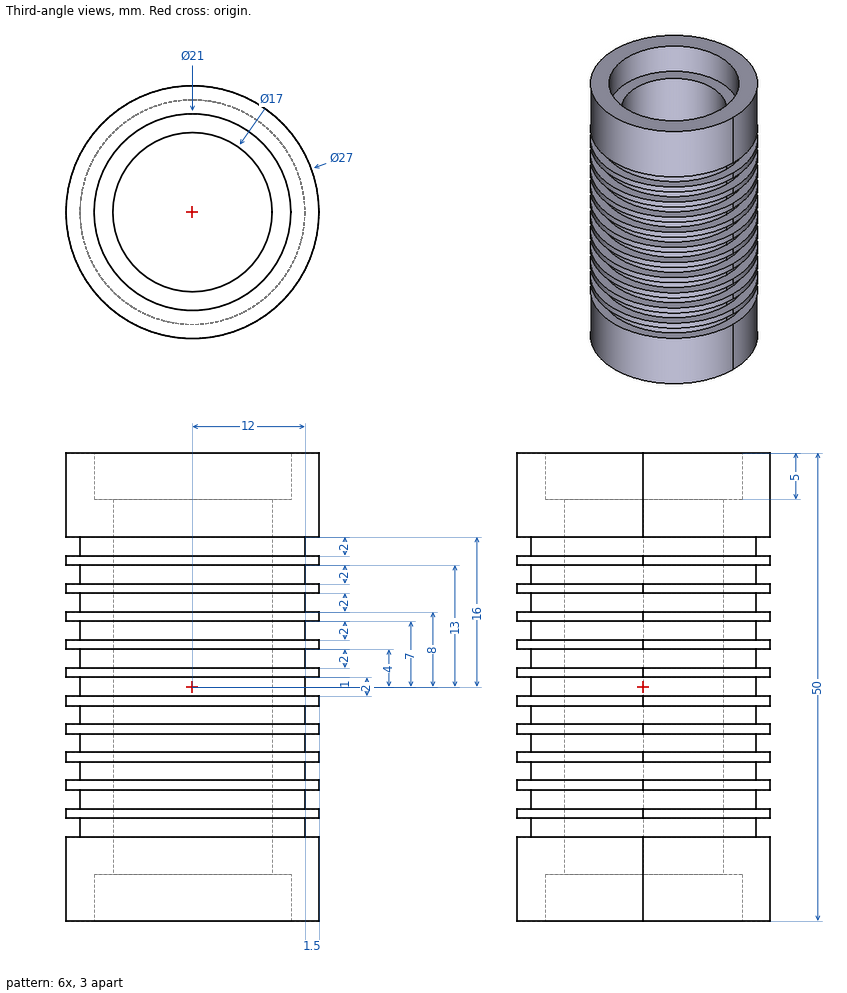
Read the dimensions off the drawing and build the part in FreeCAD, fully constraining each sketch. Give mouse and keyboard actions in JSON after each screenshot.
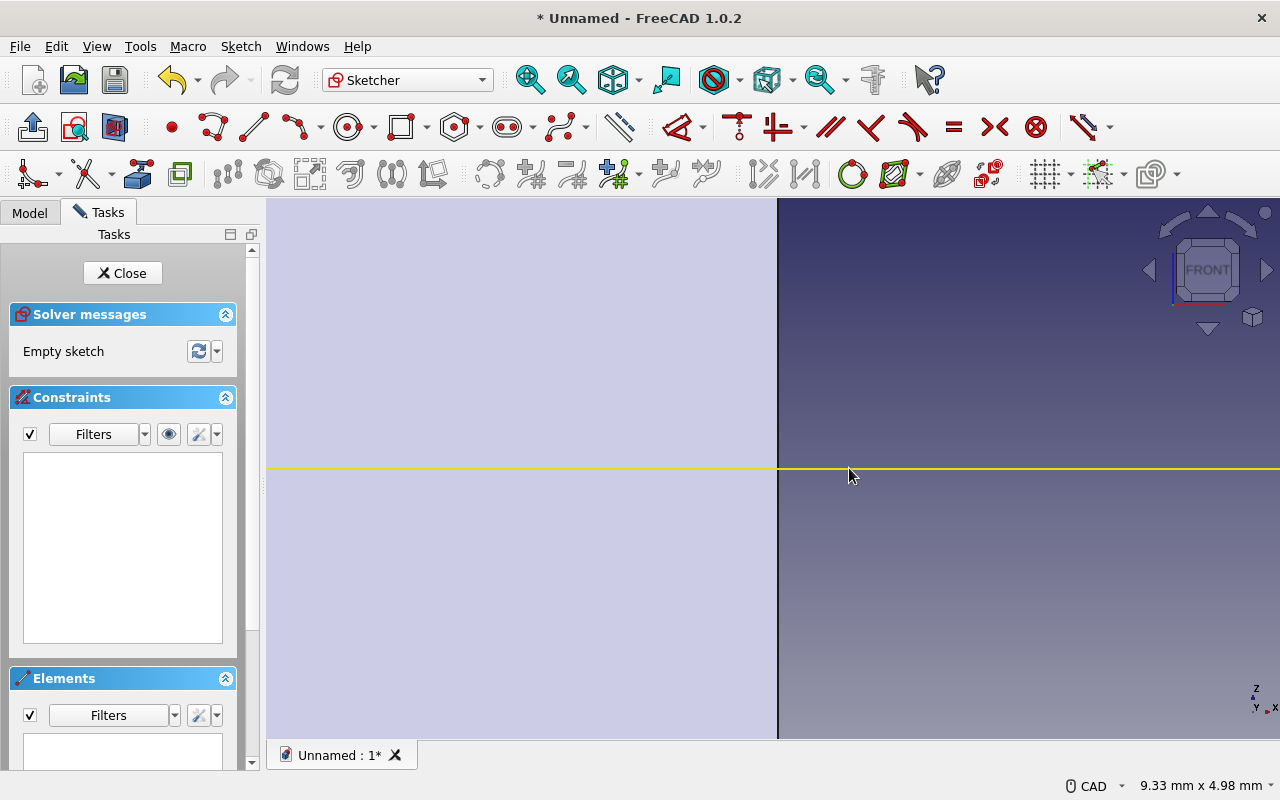
{"action": "scroll", "coordinate": [682, 469], "scroll_direction": "up", "scroll_amount": 2}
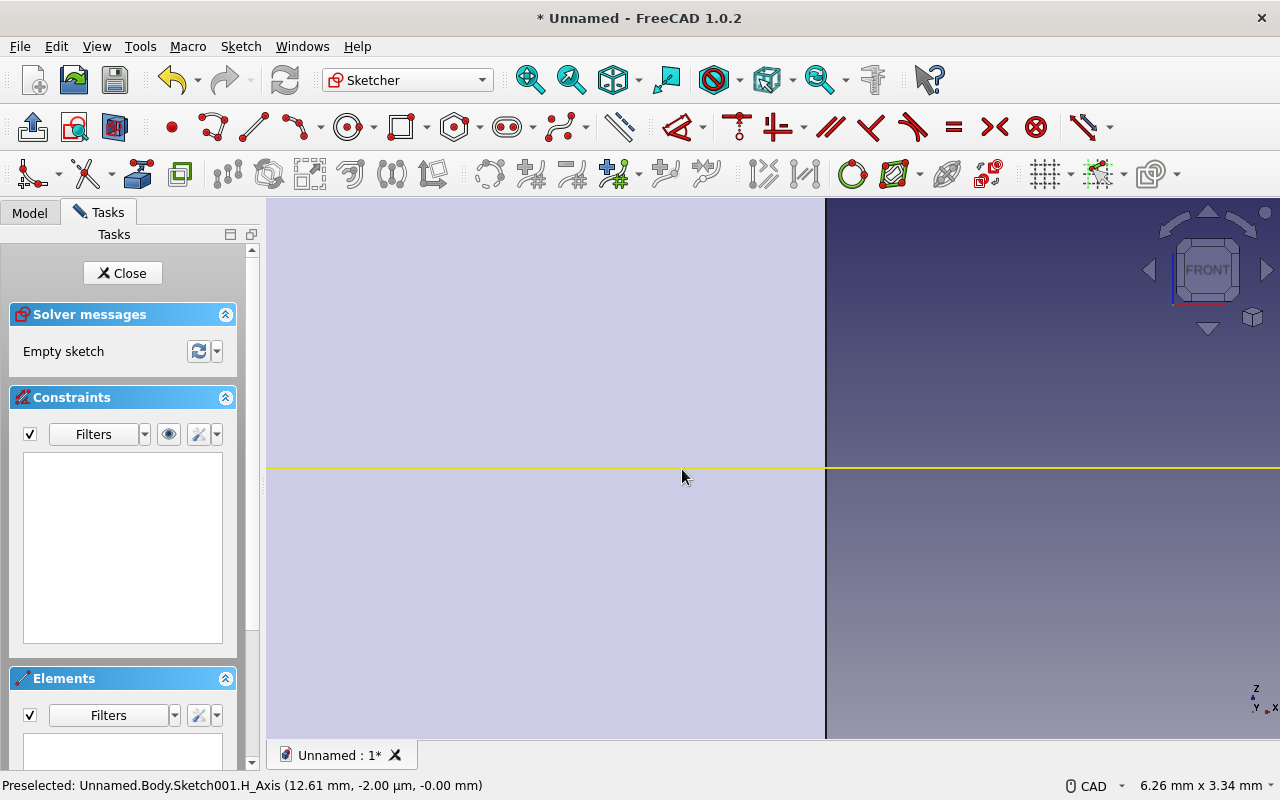
{"action": "left_click", "coordinate": [400, 128]}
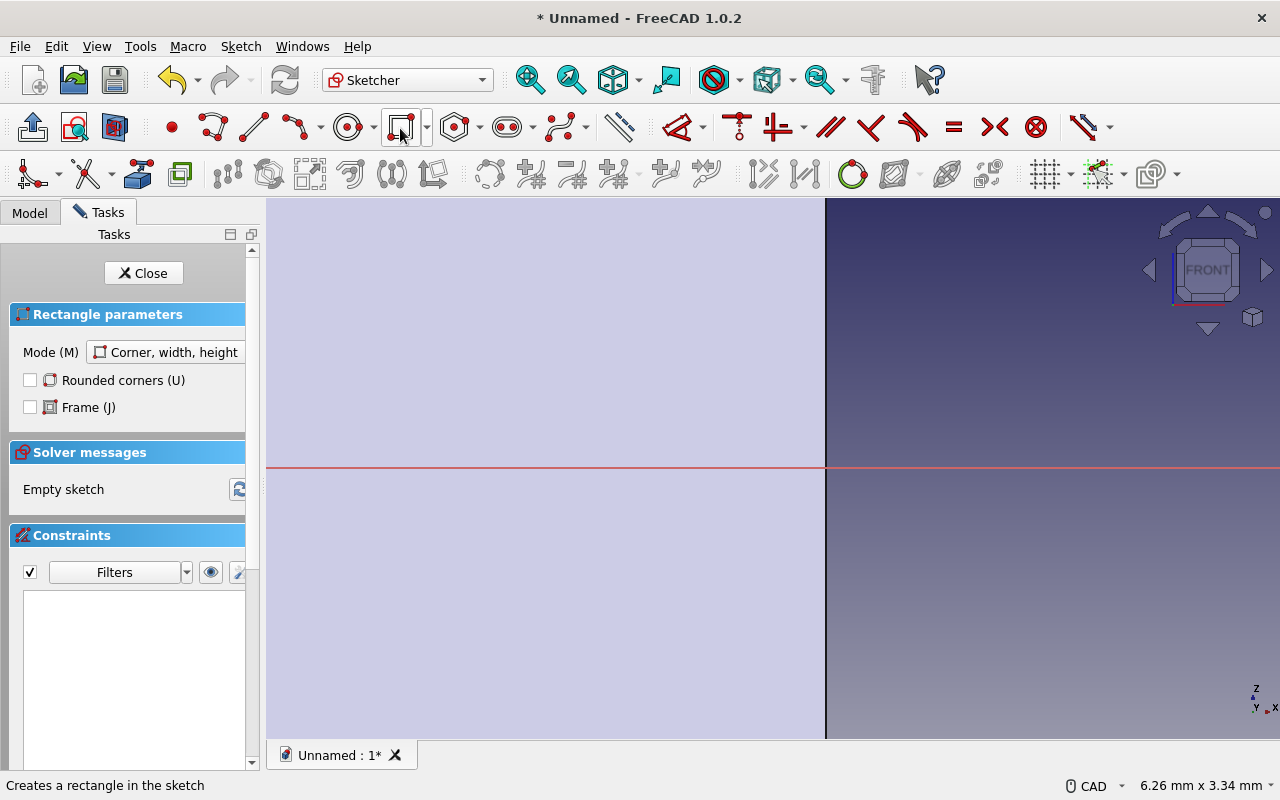
{"action": "left_click", "coordinate": [583, 306]}
{"action": "mouse_move", "coordinate": [826, 630]}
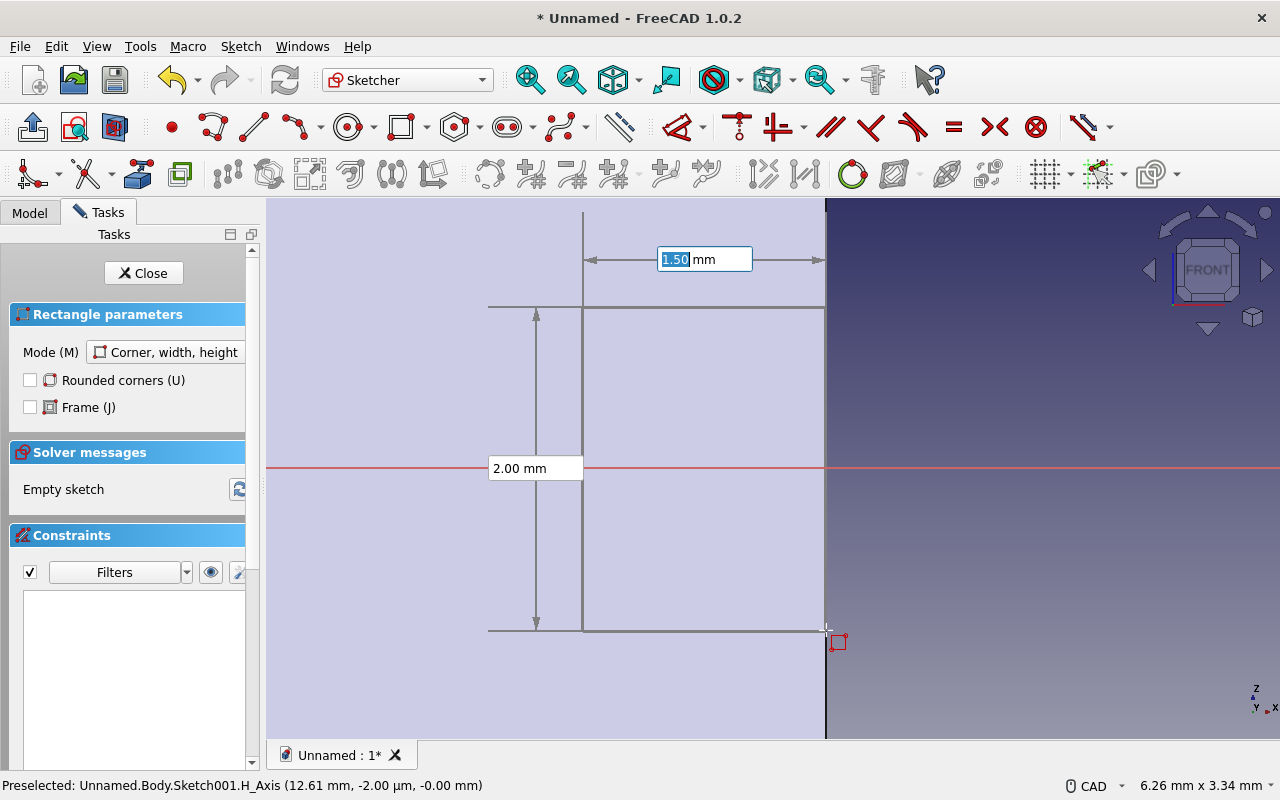
{"action": "type", "text": "1.5"}
{"action": "key", "text": "Tab"}
{"action": "type", "text": "2"}
{"action": "key", "text": "Return"}
{"action": "key", "text": "Escape"}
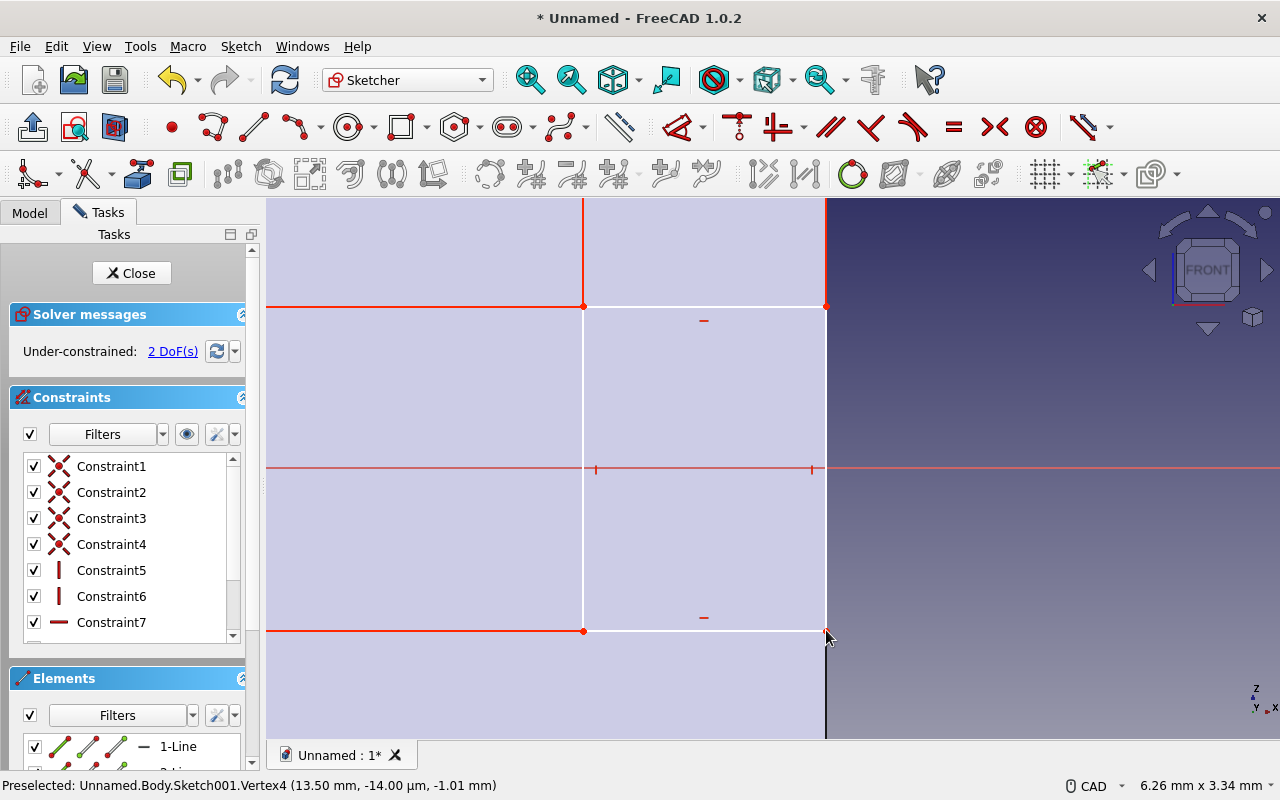
{"action": "key", "text": "d"}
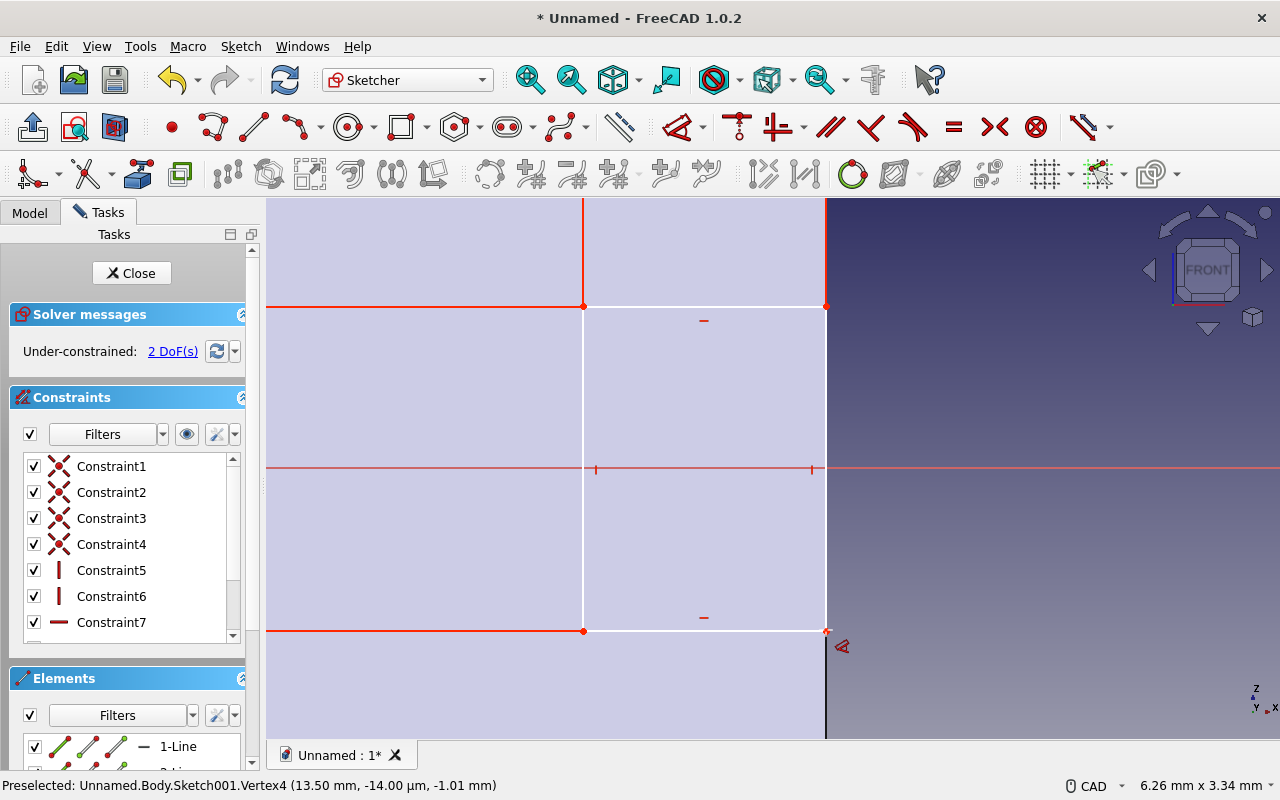
{"action": "left_click", "coordinate": [583, 307]}
{"action": "left_click", "coordinate": [617, 388]}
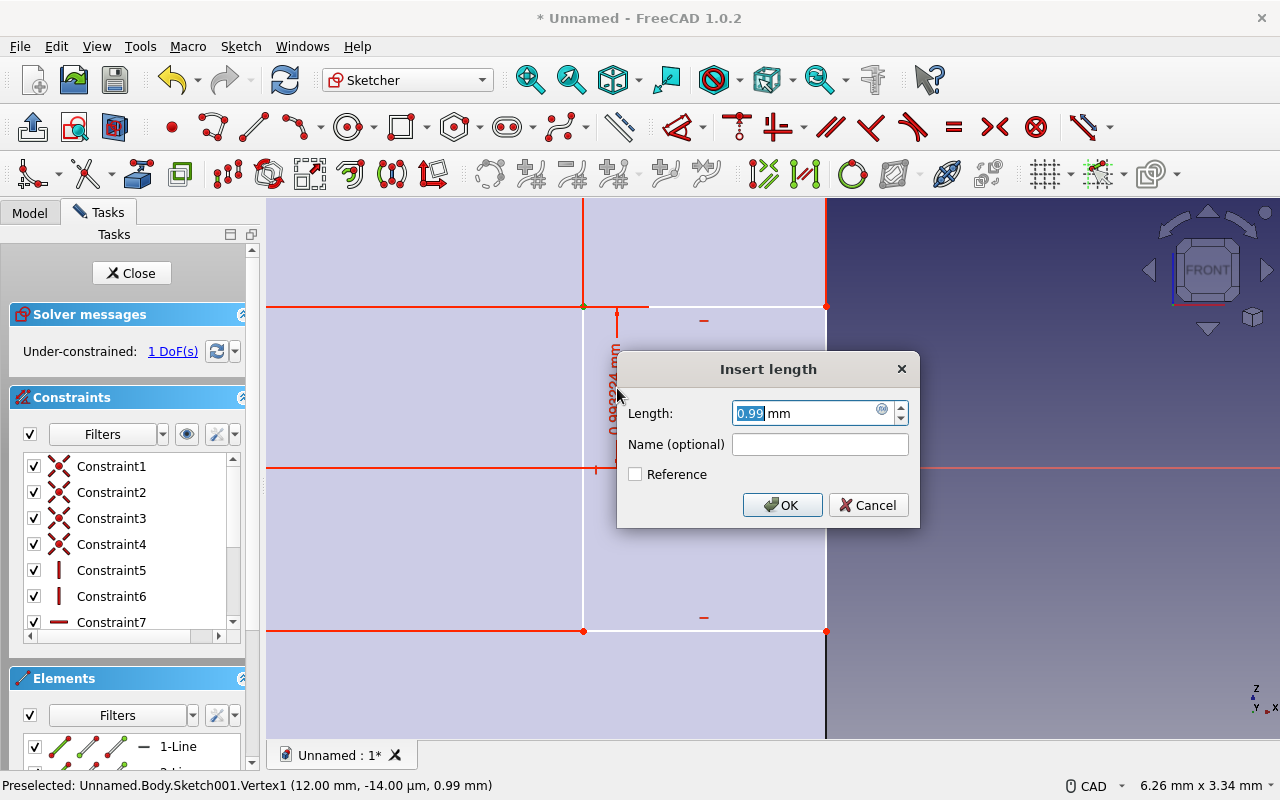
{"action": "type", "text": "1"}
{"action": "key", "text": "Return"}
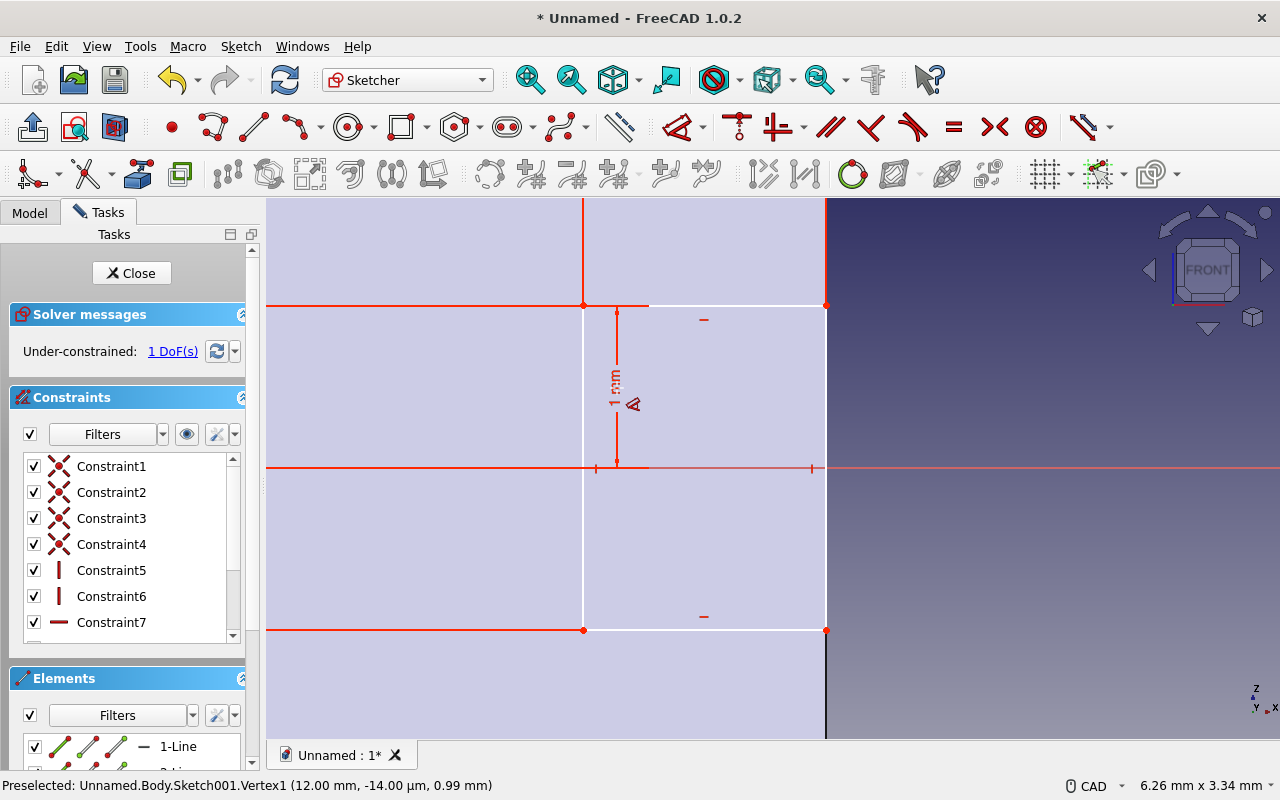
{"action": "left_click", "coordinate": [583, 306]}
{"action": "left_click", "coordinate": [438, 272]}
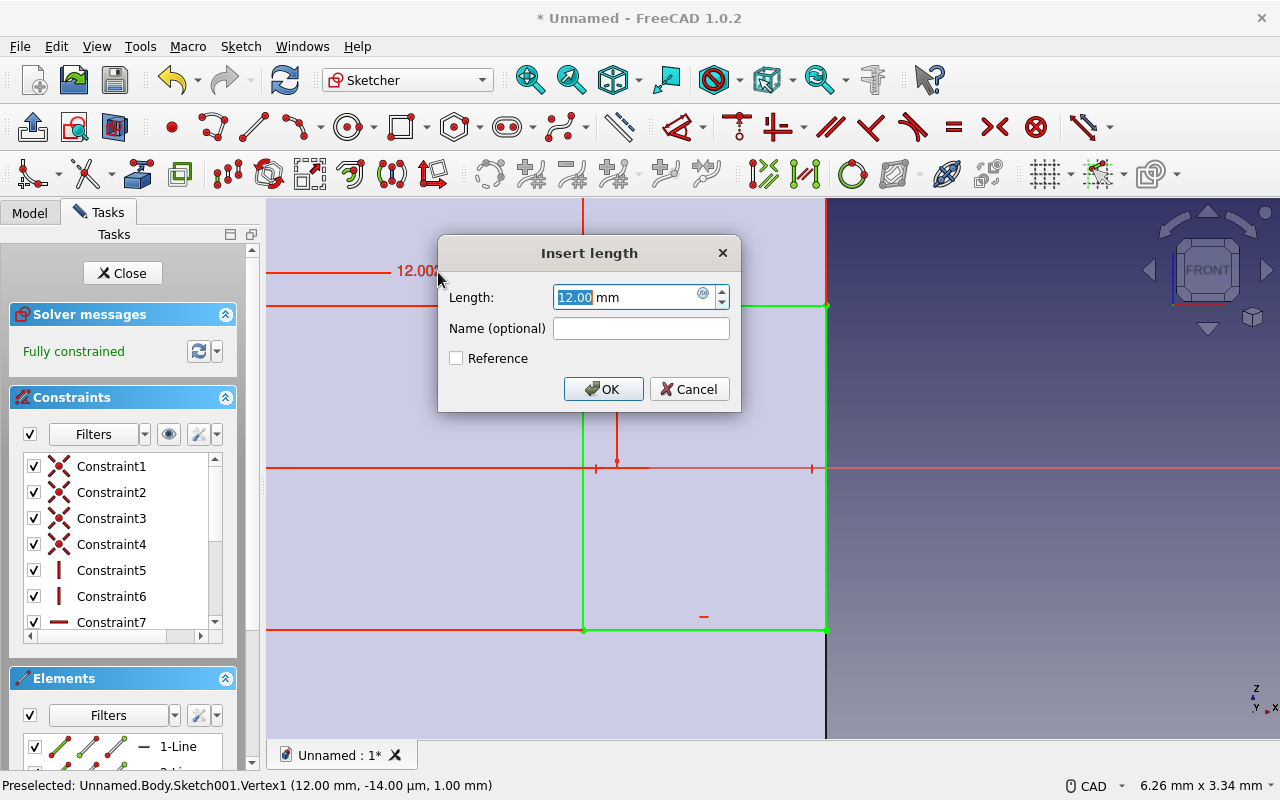
{"action": "type", "text": "12"}
{"action": "key", "text": "Return"}
{"action": "key", "text": "Escape"}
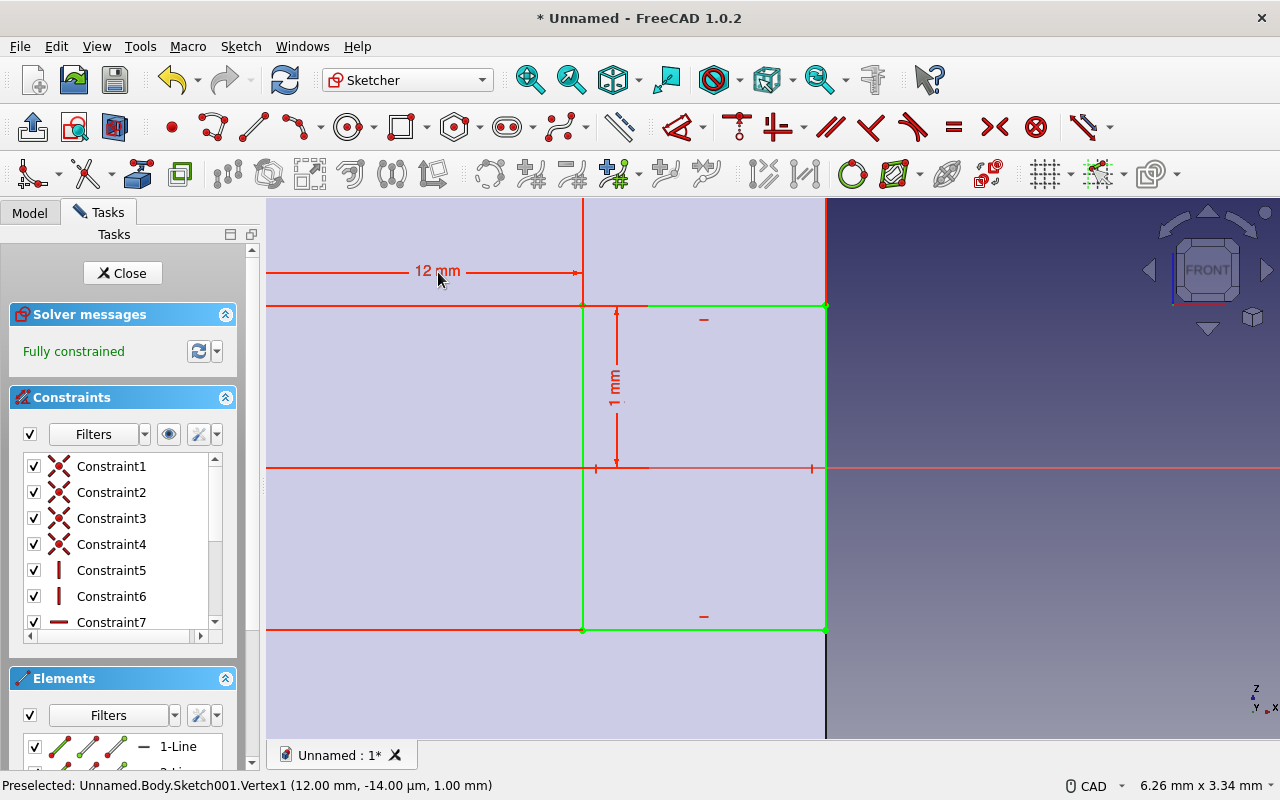
{"action": "left_click", "coordinate": [123, 273]}